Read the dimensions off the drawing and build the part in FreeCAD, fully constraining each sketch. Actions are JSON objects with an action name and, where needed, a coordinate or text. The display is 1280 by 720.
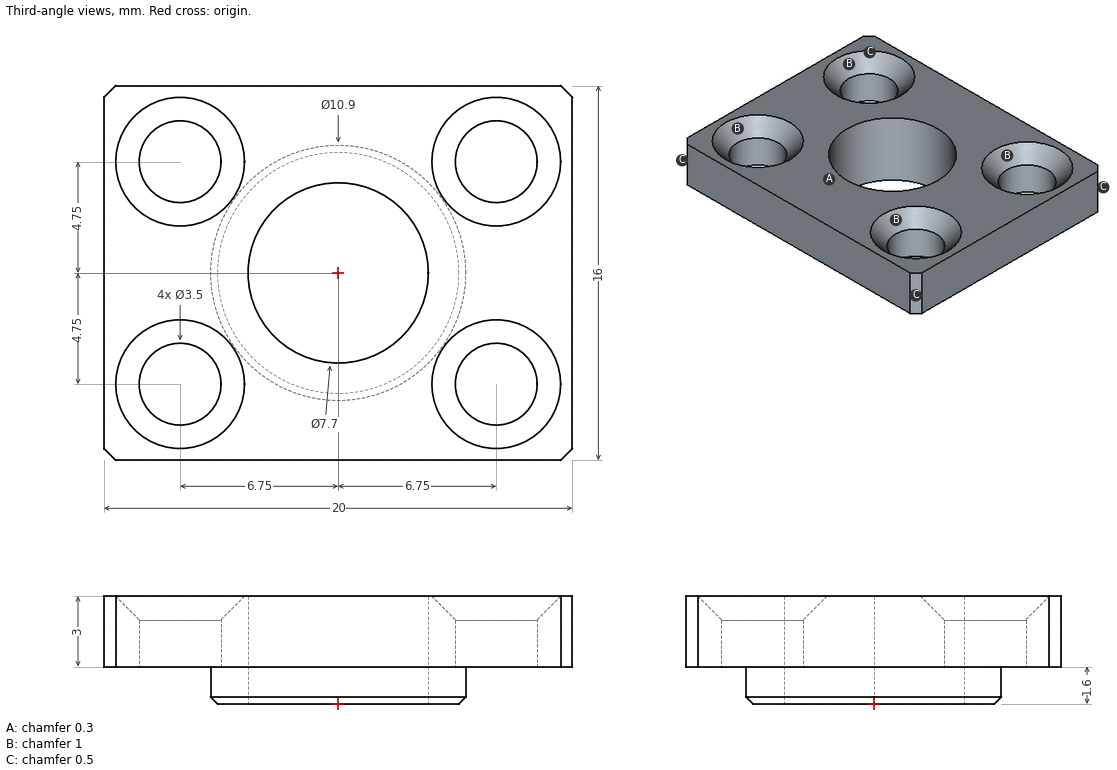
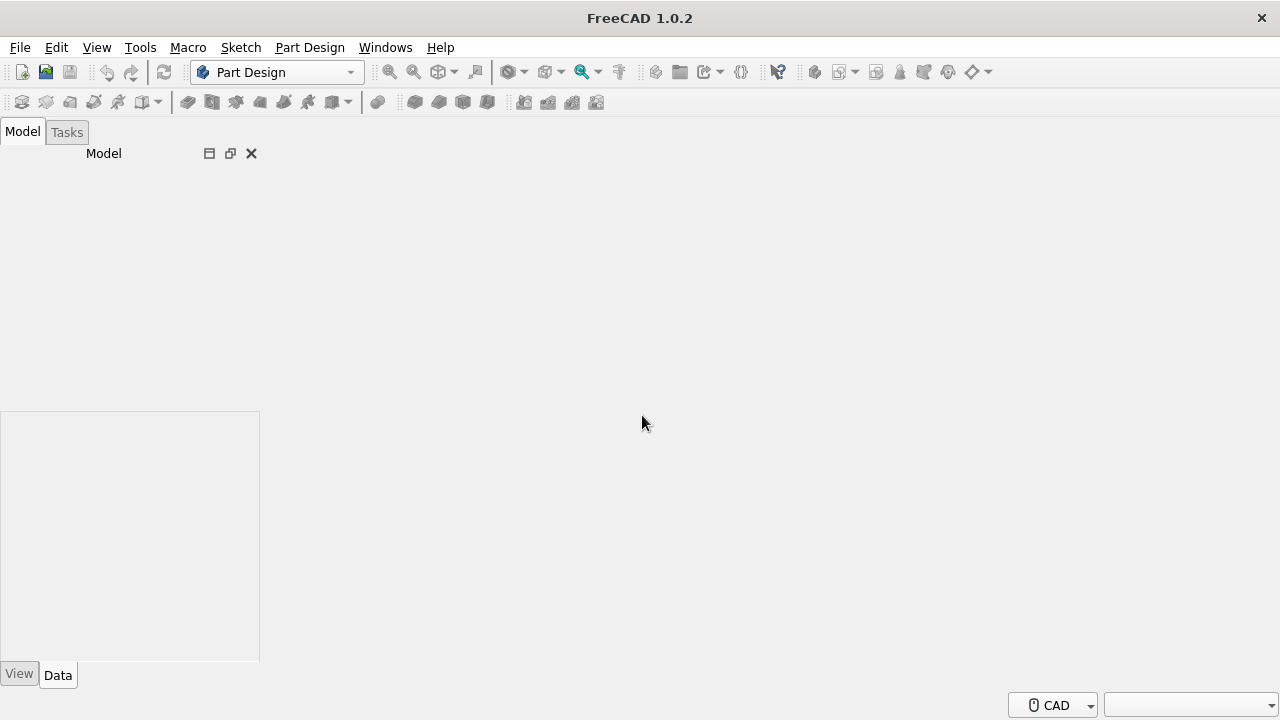
{"action": "key", "text": "ctrl+n"}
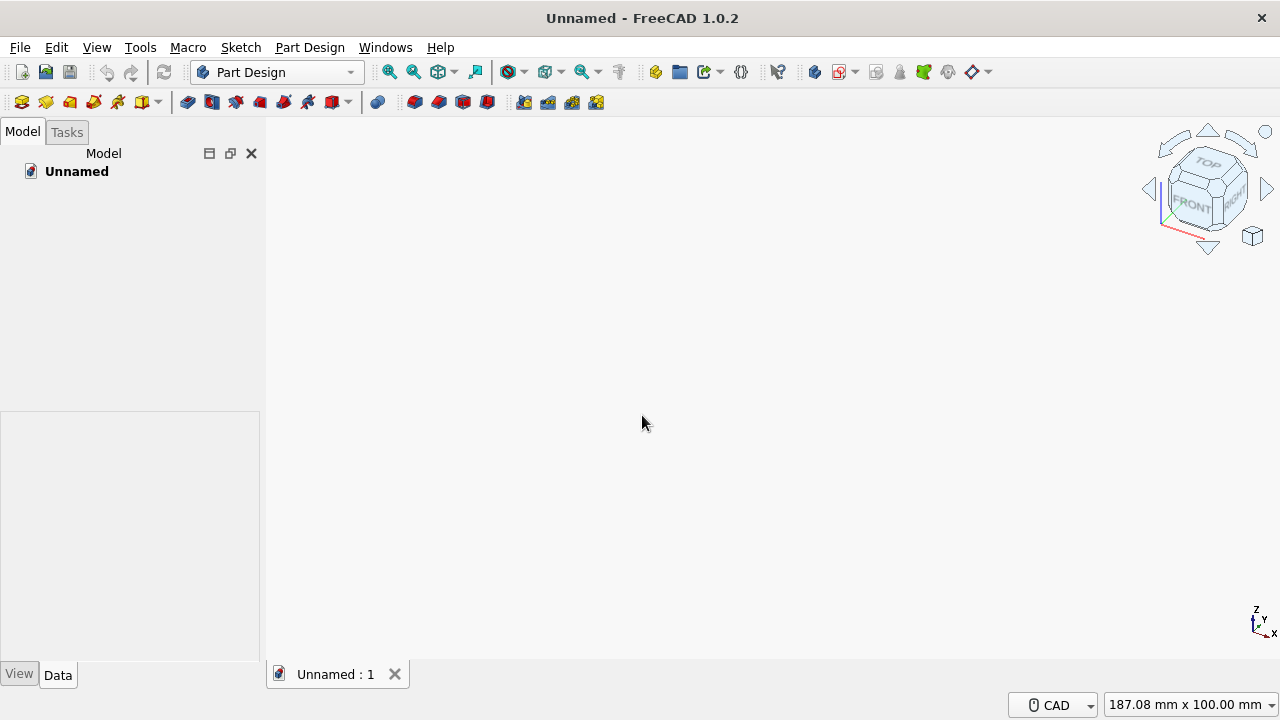
{"action": "left_click", "coordinate": [840, 72]}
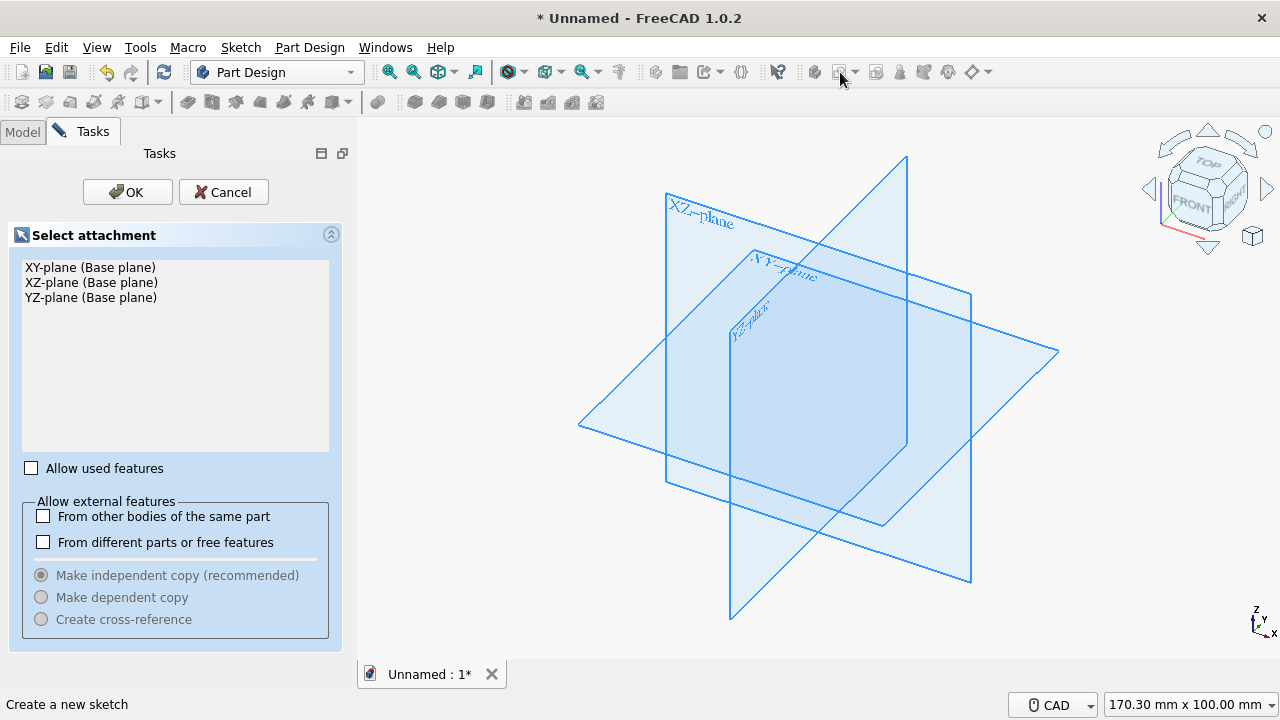
{"action": "left_click", "coordinate": [82, 268]}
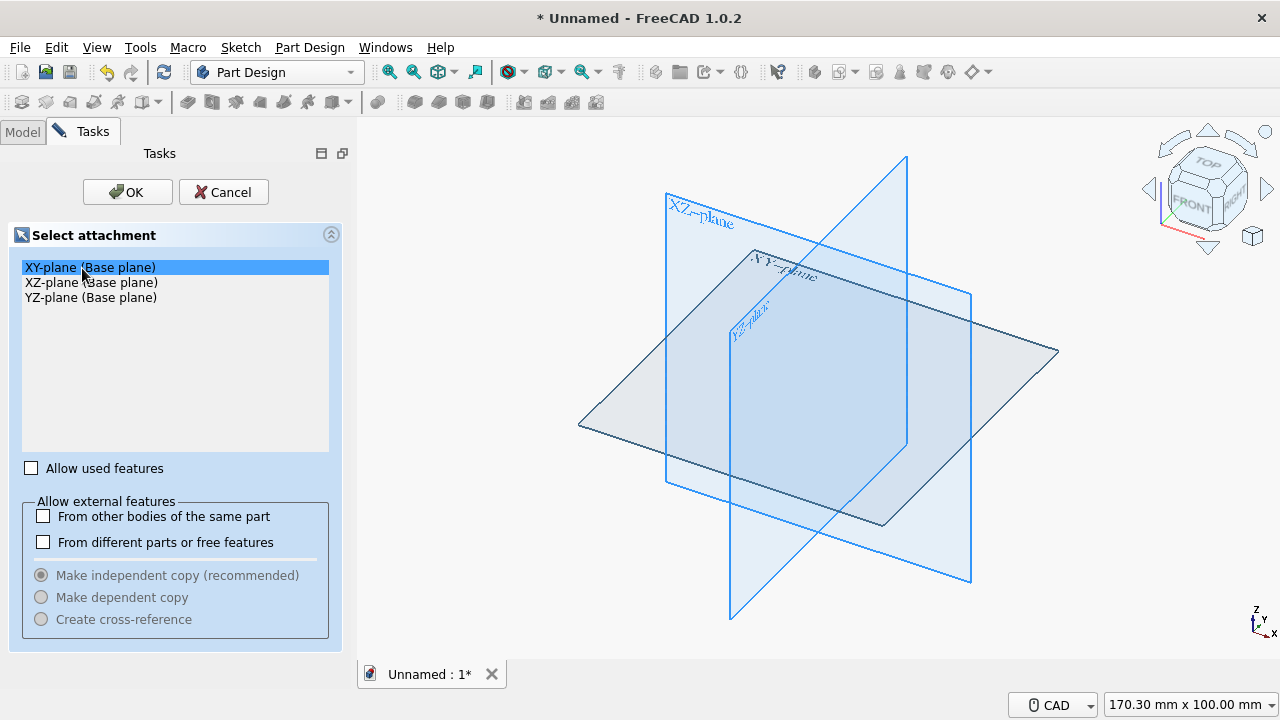
{"action": "left_click", "coordinate": [128, 192]}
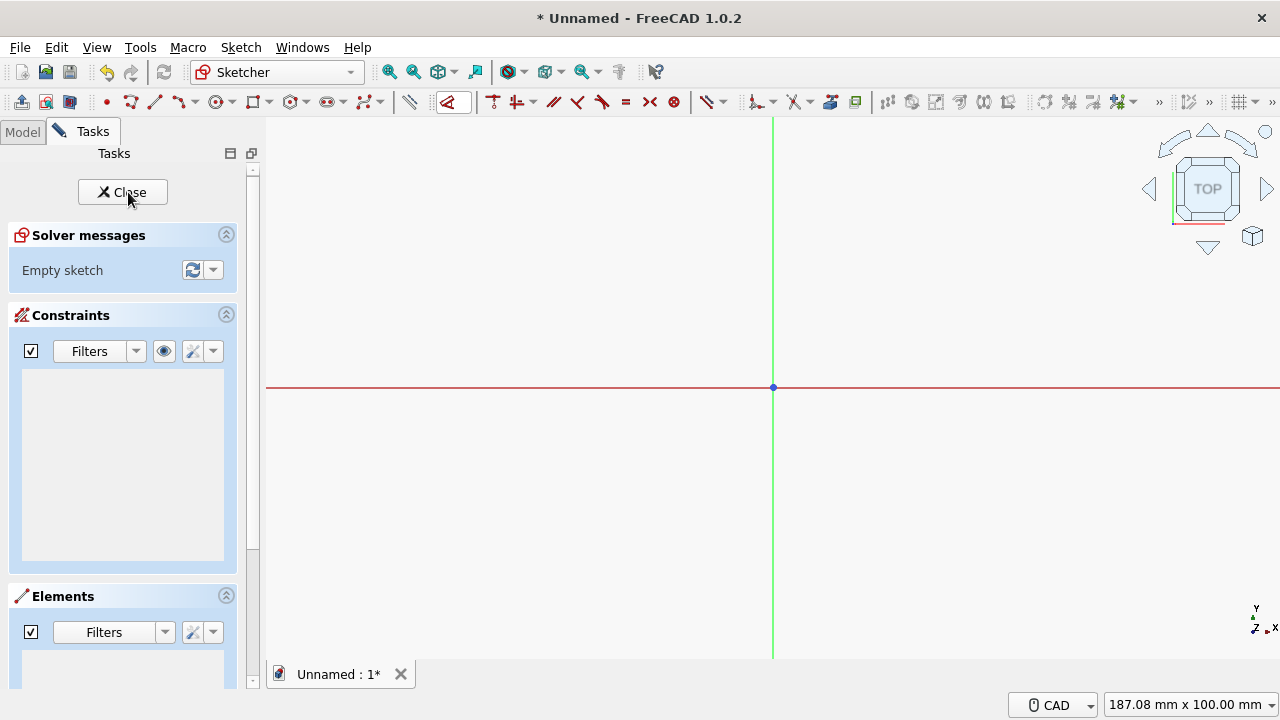
{"action": "scroll", "coordinate": [787, 388], "scroll_direction": "up", "scroll_amount": 9}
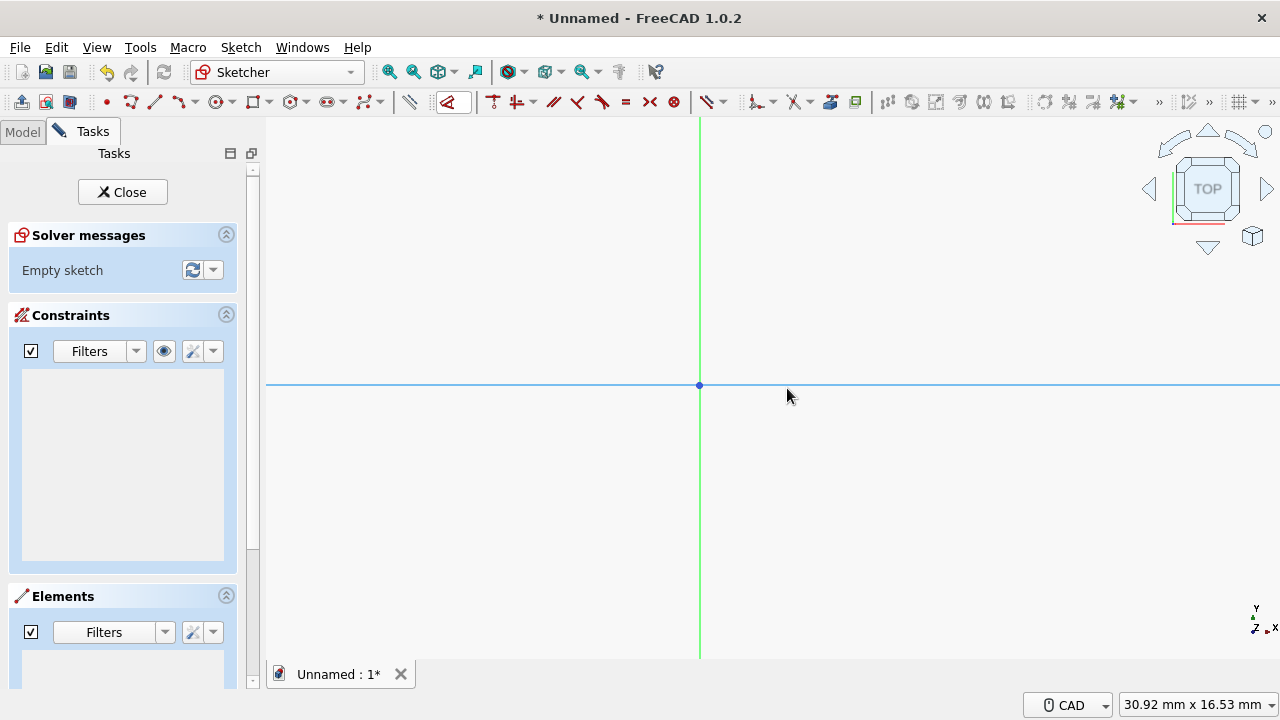
{"action": "key", "text": "g c"}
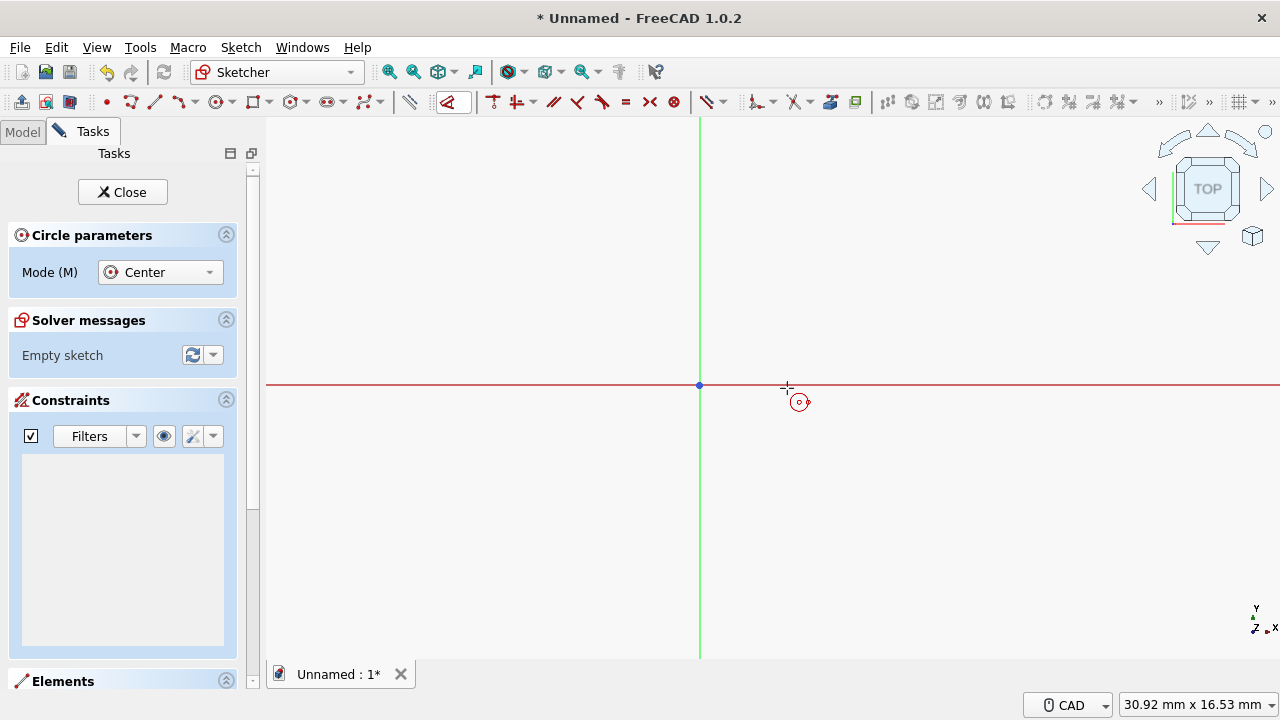
{"action": "left_click", "coordinate": [700, 385]}
{"action": "left_click", "coordinate": [826, 259]}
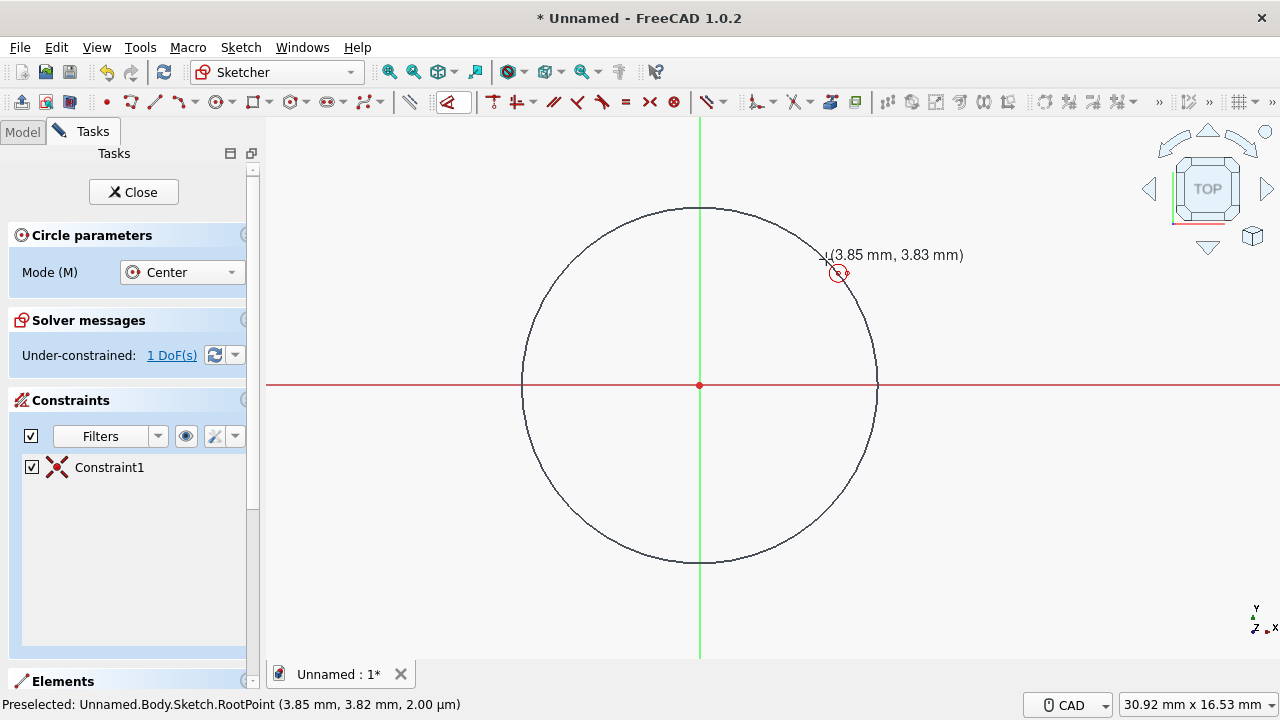
{"action": "left_click", "coordinate": [700, 385]}
{"action": "left_click", "coordinate": [789, 296]}
{"action": "key", "text": "Escape"}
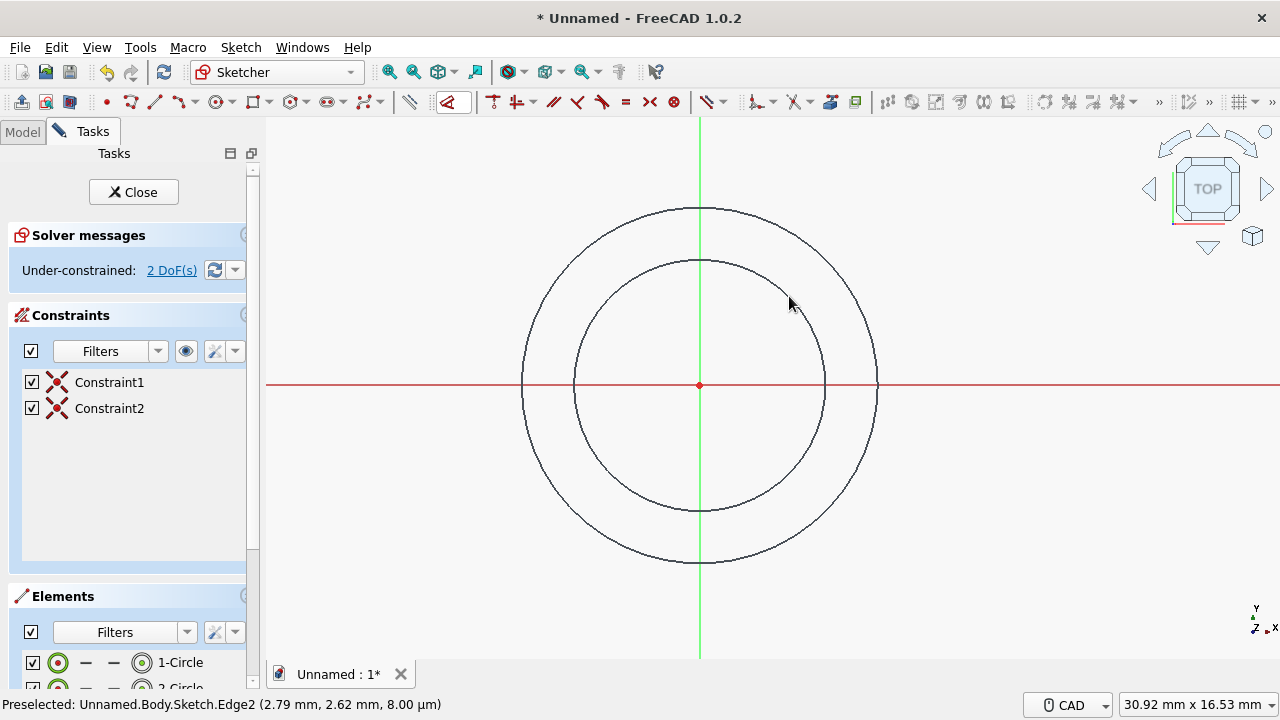
{"action": "left_click", "coordinate": [825, 259]}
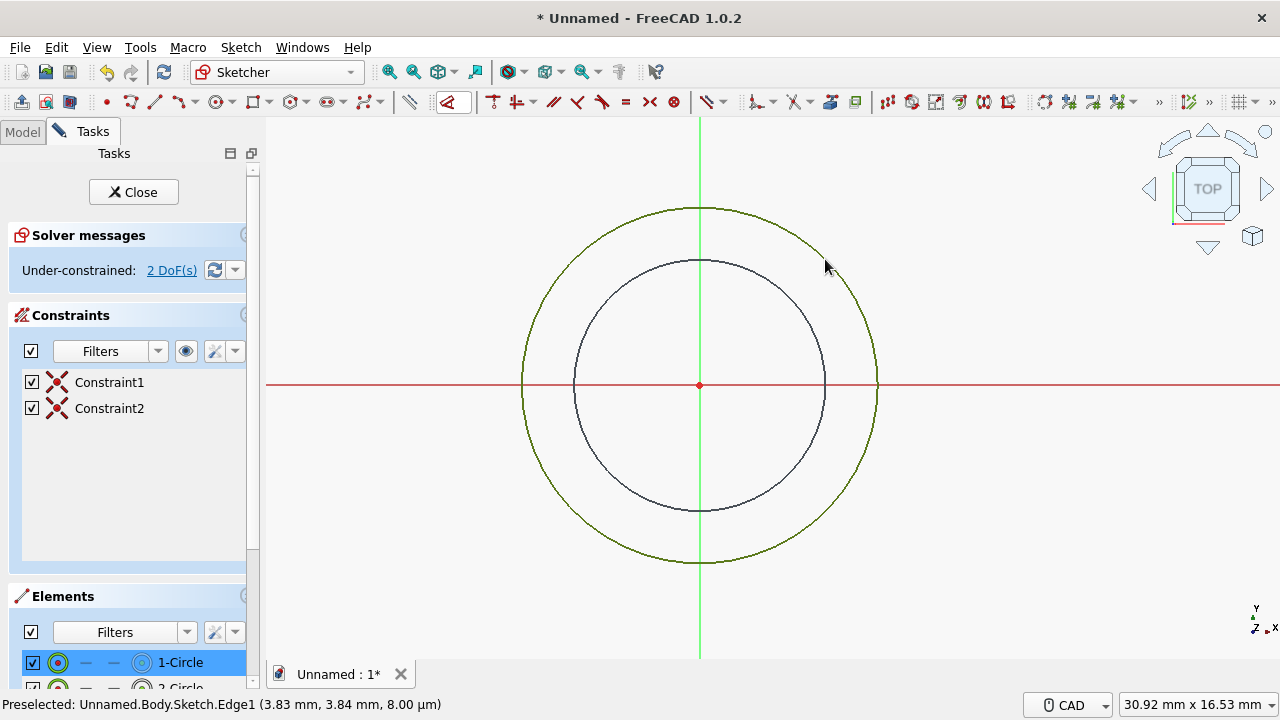
{"action": "key", "text": "k o"}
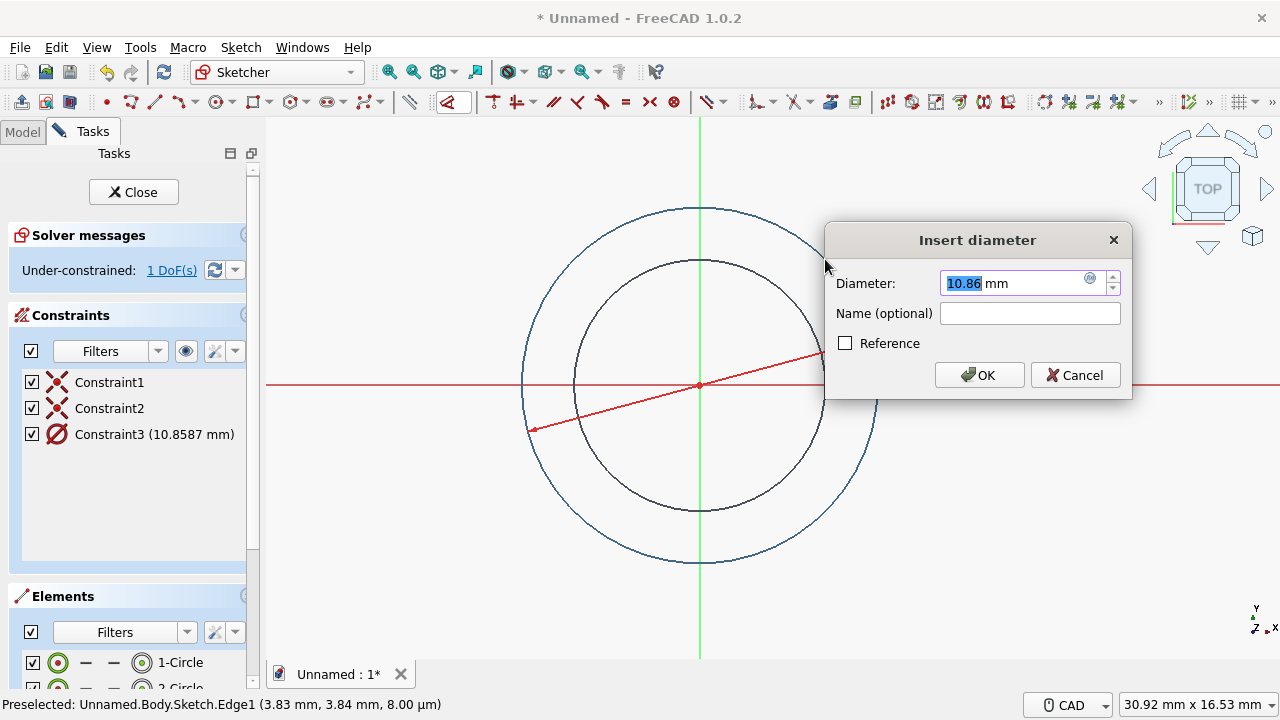
{"action": "type", "text": "10.9"}
{"action": "key", "text": "Return"}